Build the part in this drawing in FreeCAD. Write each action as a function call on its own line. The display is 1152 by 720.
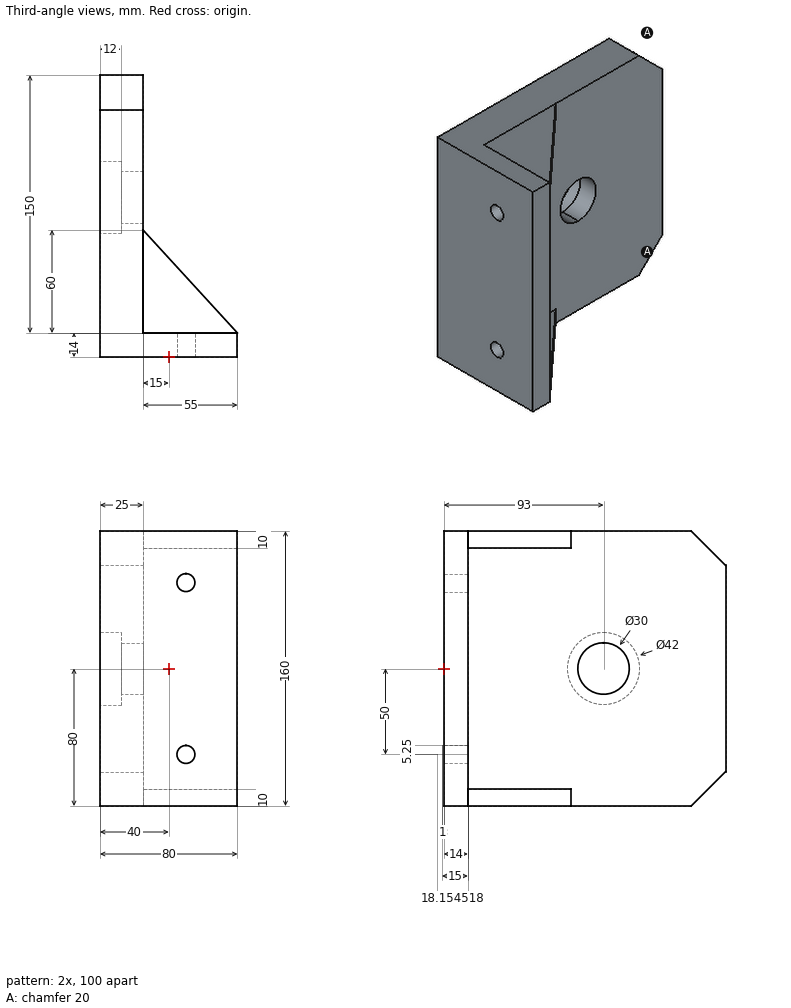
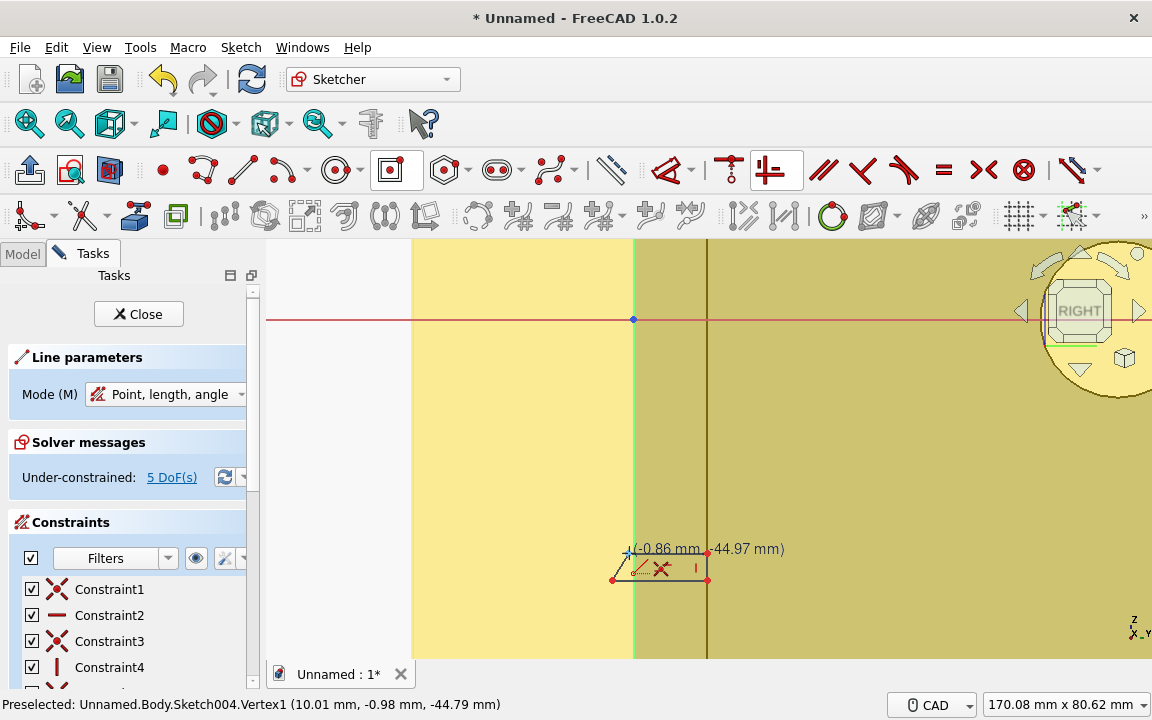
scroll(603, 580, up, 3)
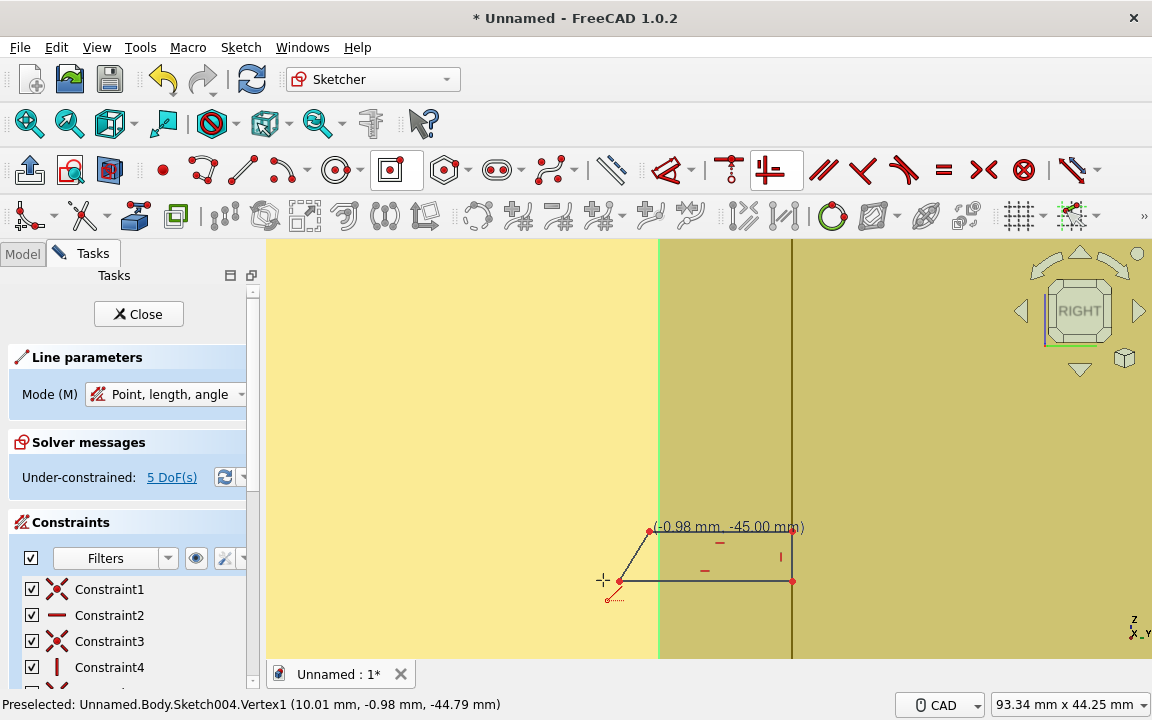
click(602, 579)
click(550, 579)
key(Escape)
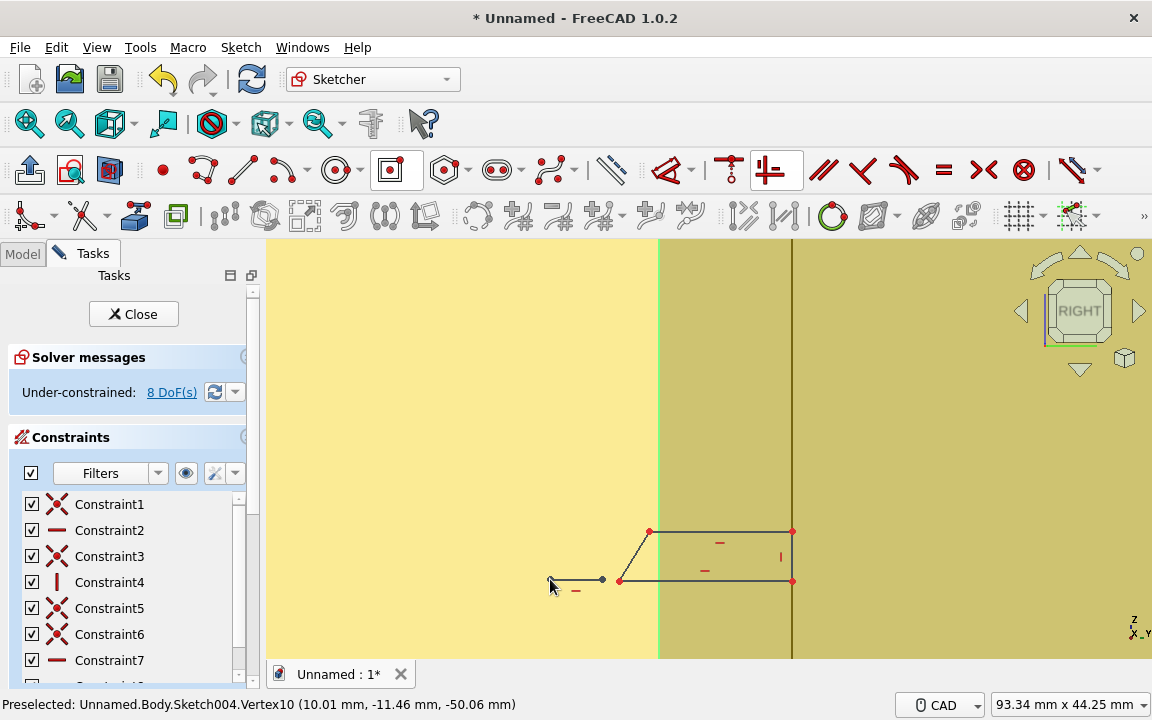
click(586, 580)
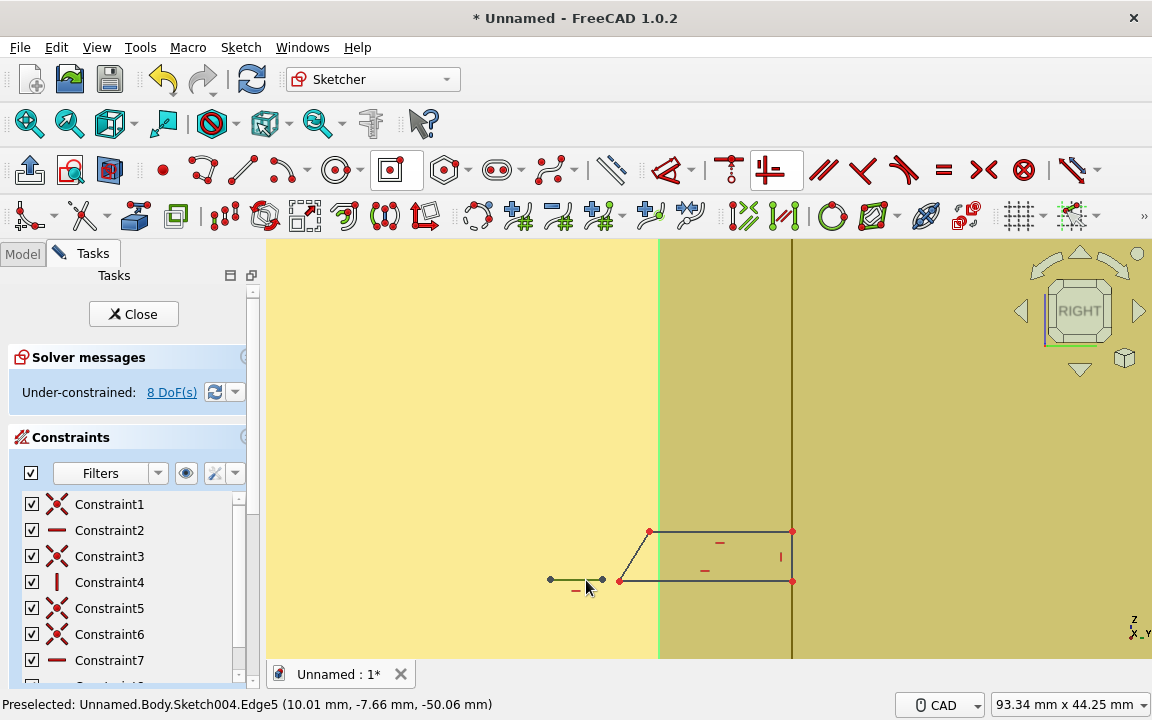
click(612, 170)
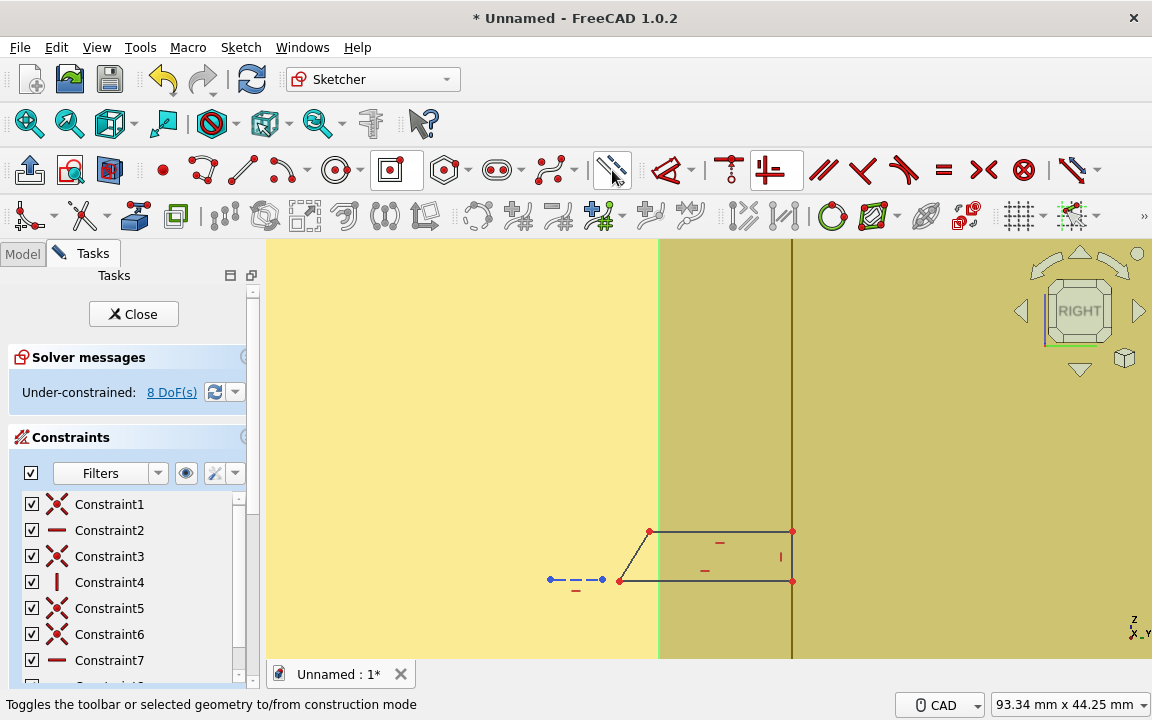
click(666, 170)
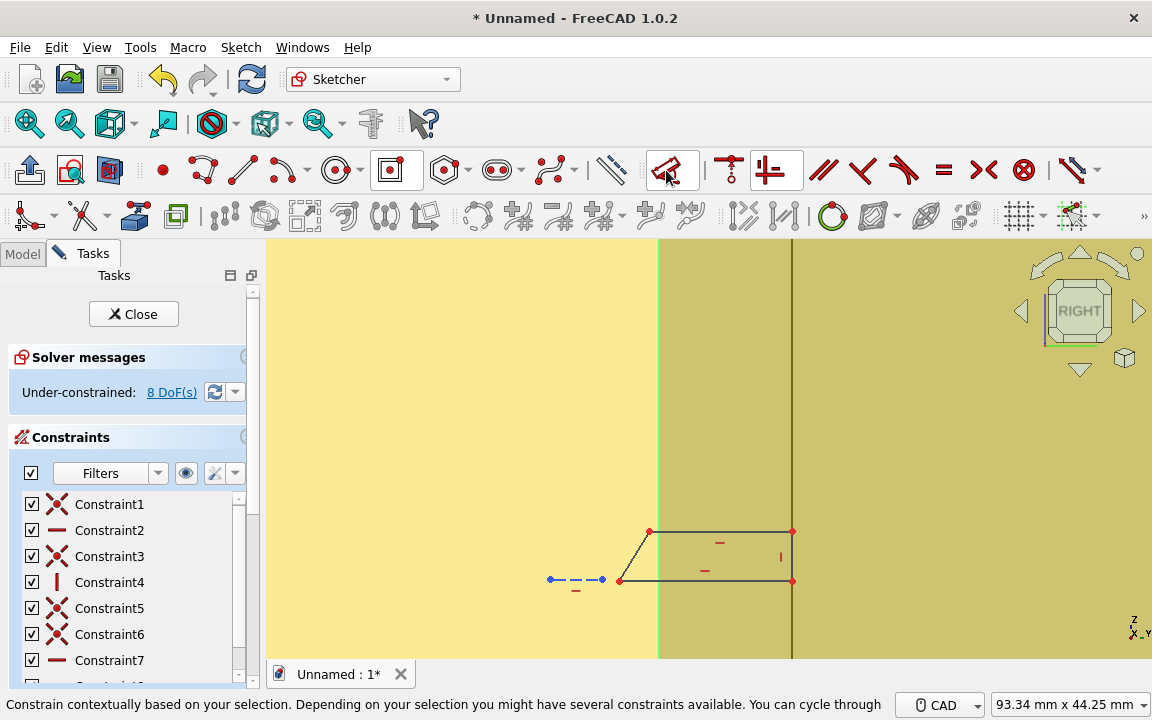
click(749, 532)
click(721, 566)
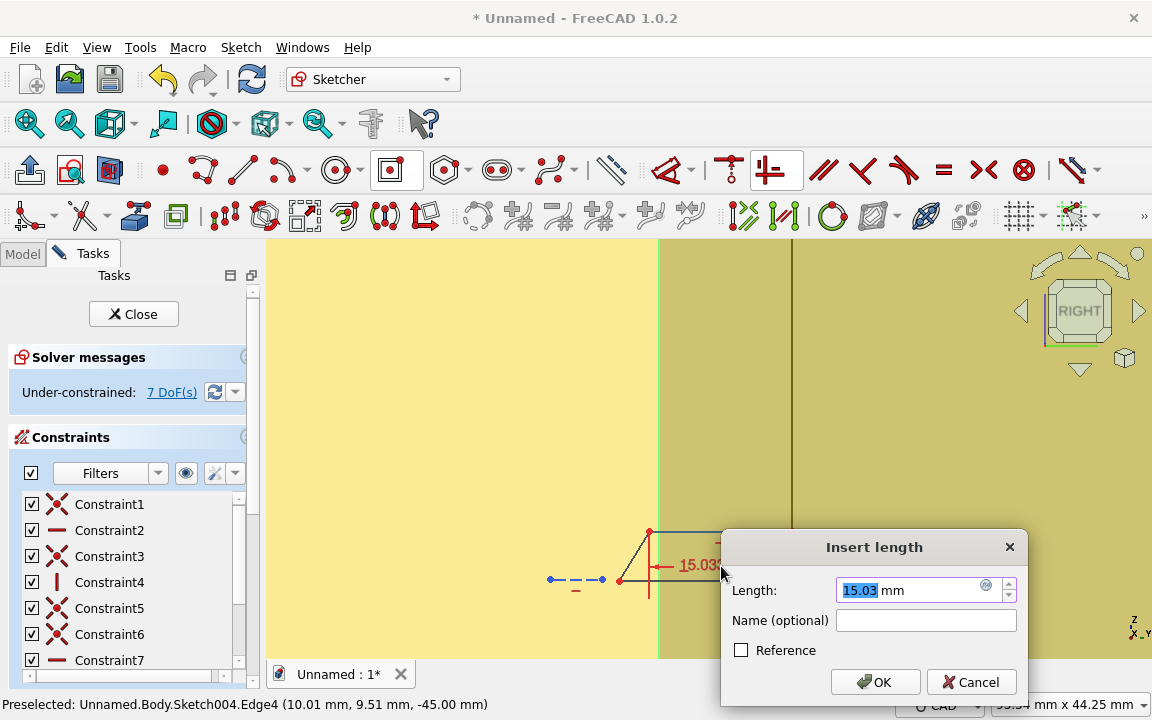
text(15)
key(Return)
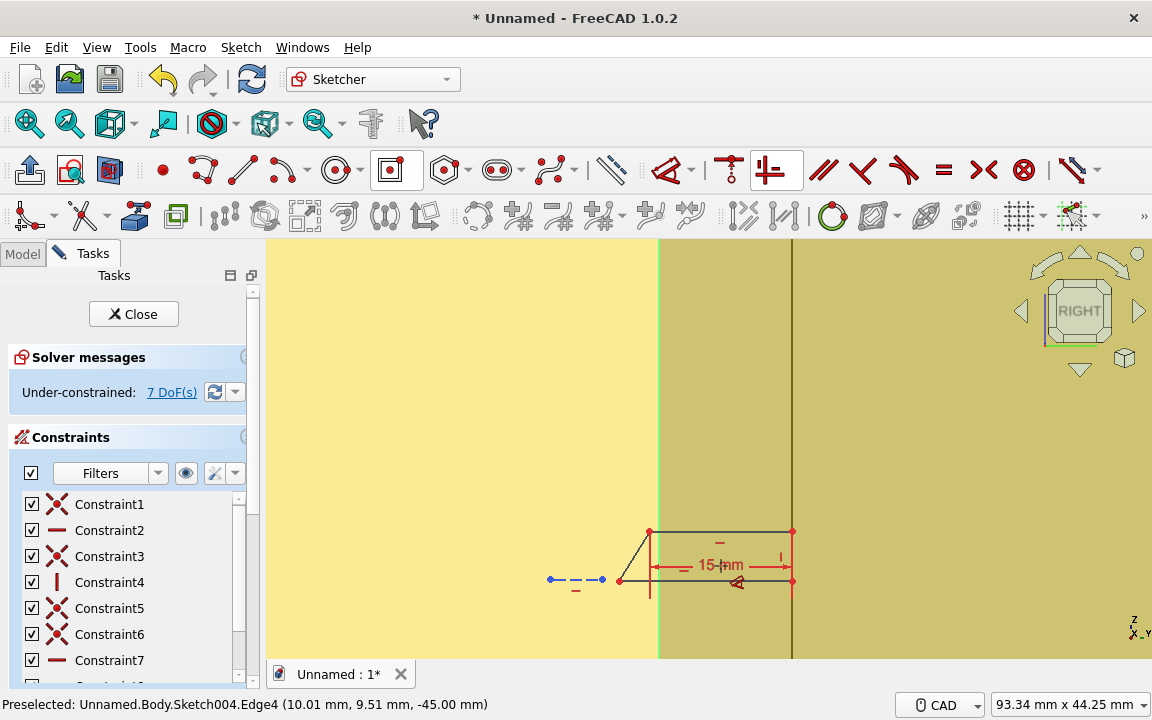
scroll(650, 532, up, 8)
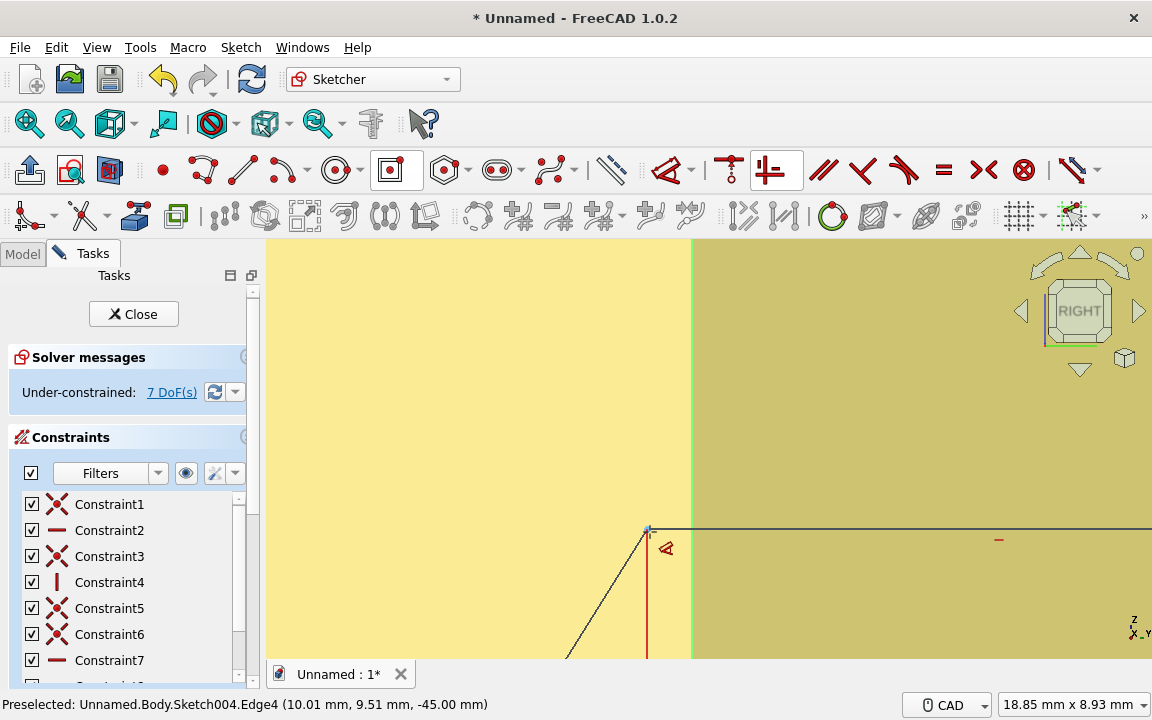
click(647, 529)
click(669, 563)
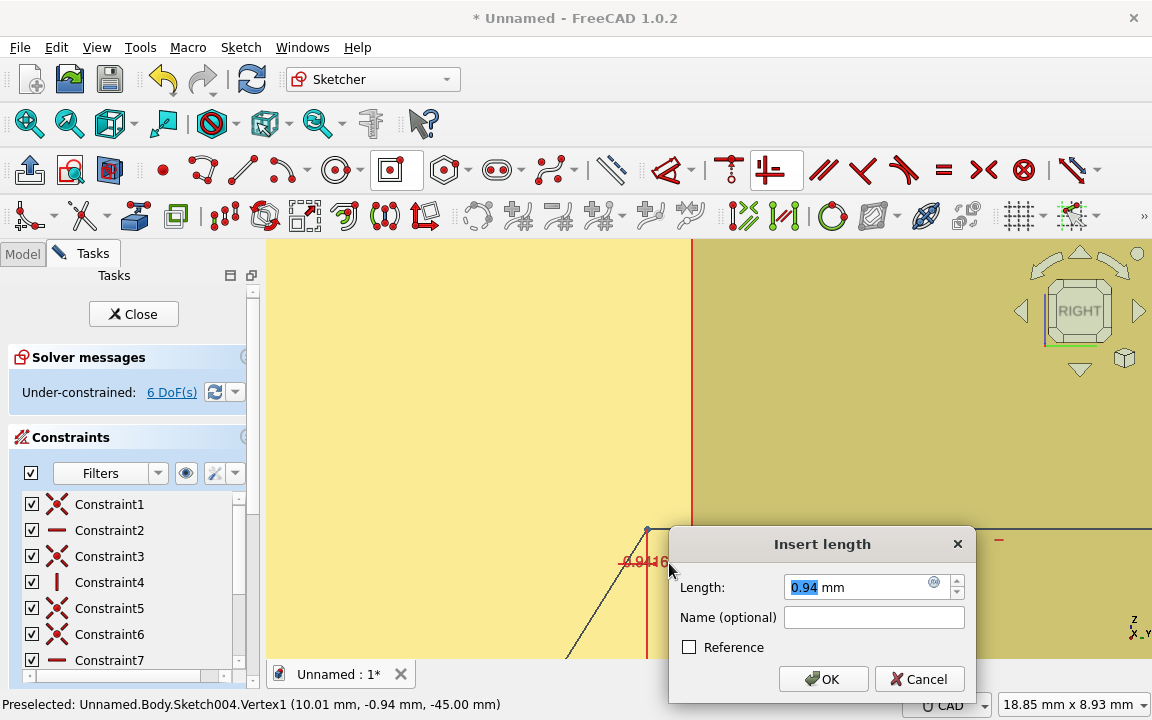
text(1)
key(Return)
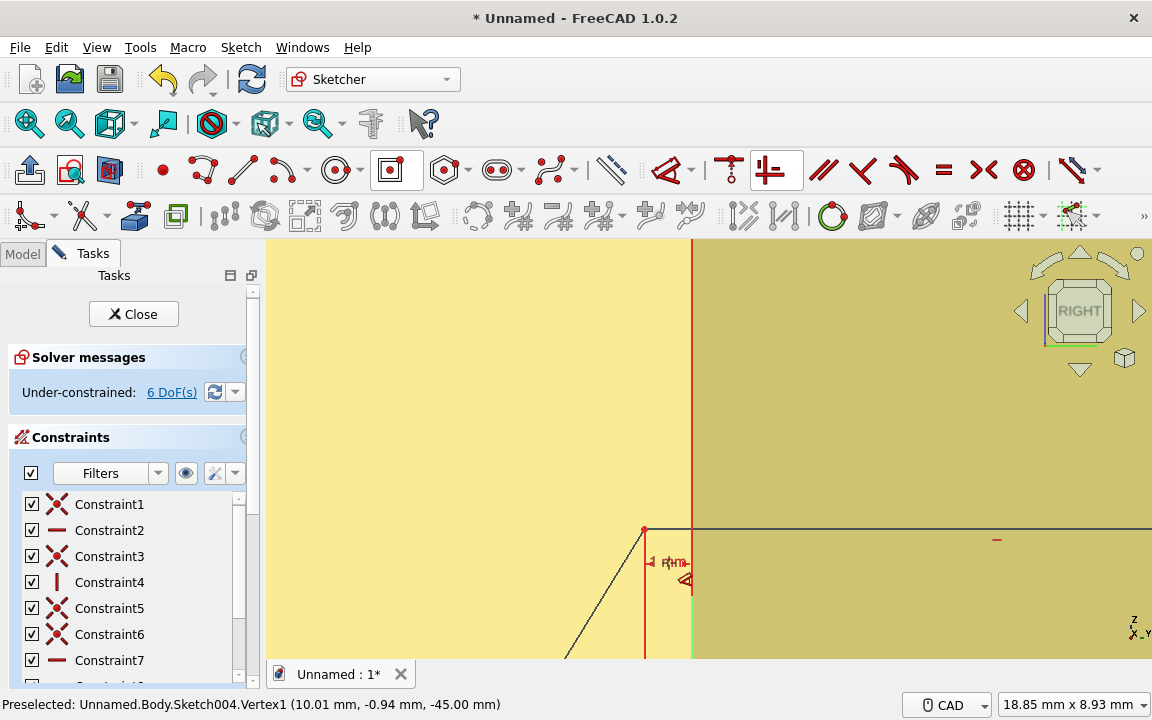
scroll(627, 556, down, 11)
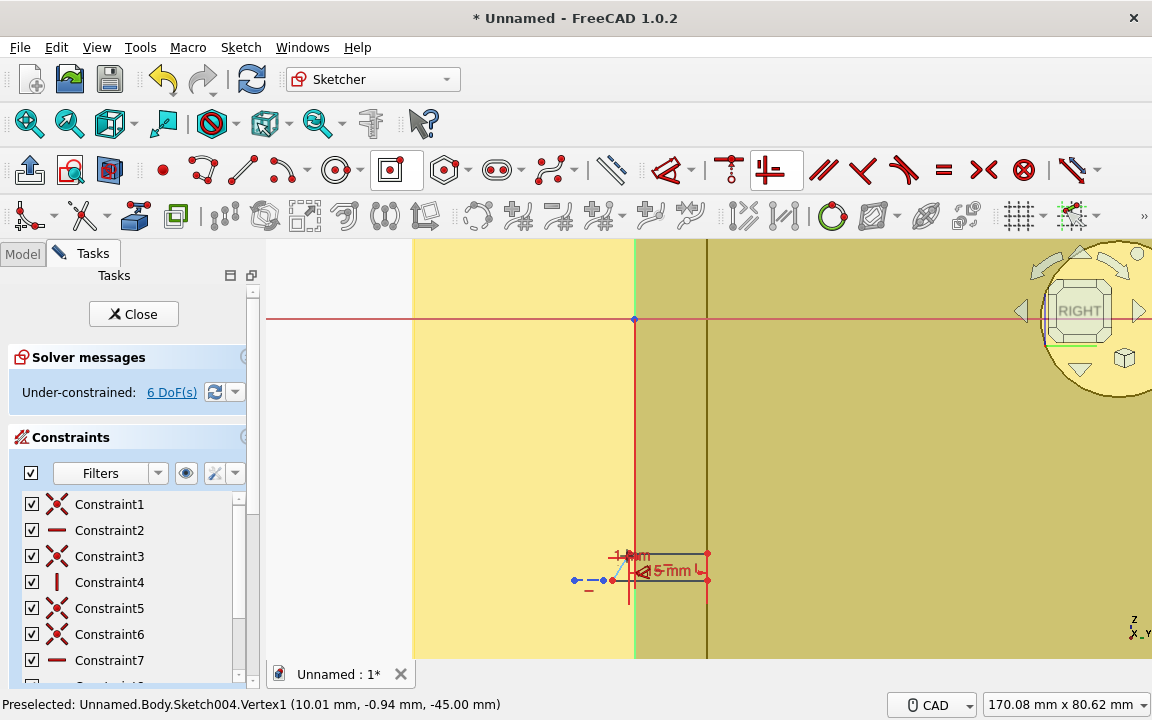
scroll(613, 581, up, 2)